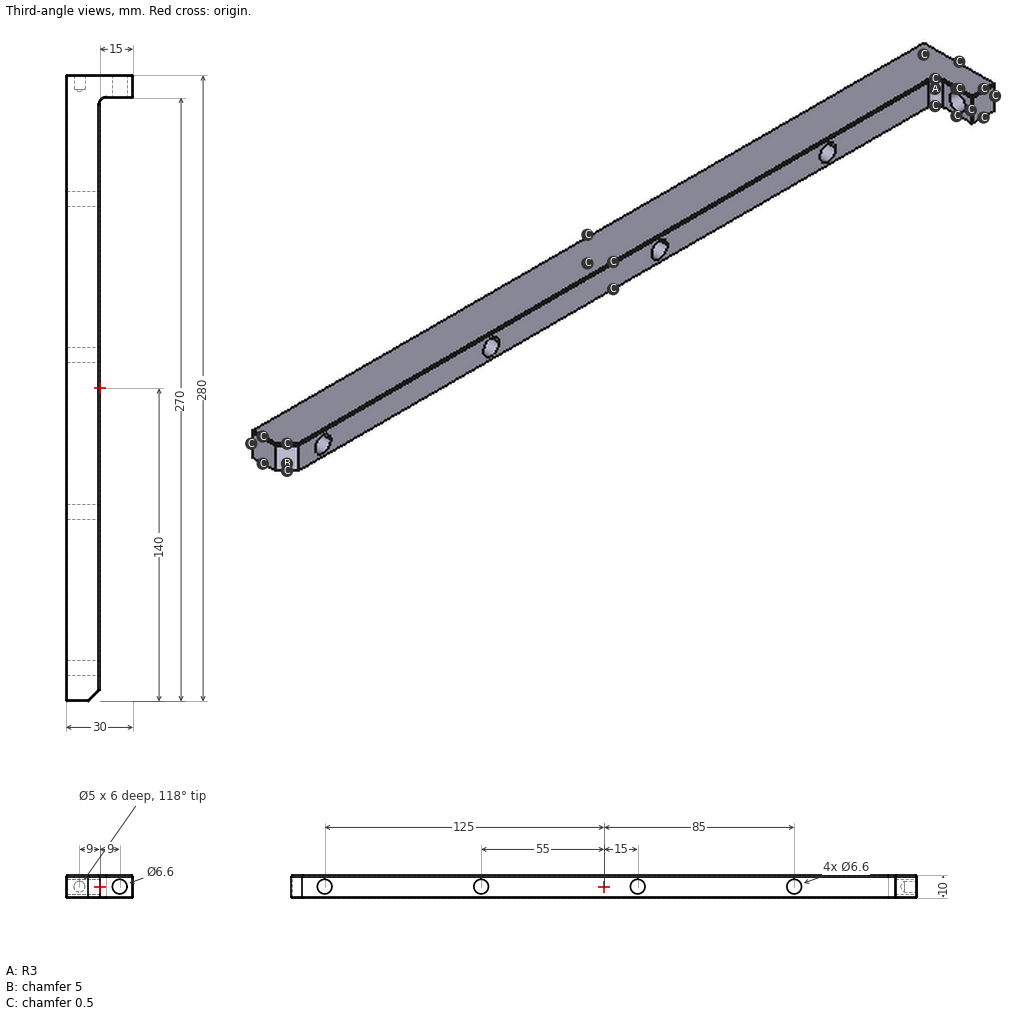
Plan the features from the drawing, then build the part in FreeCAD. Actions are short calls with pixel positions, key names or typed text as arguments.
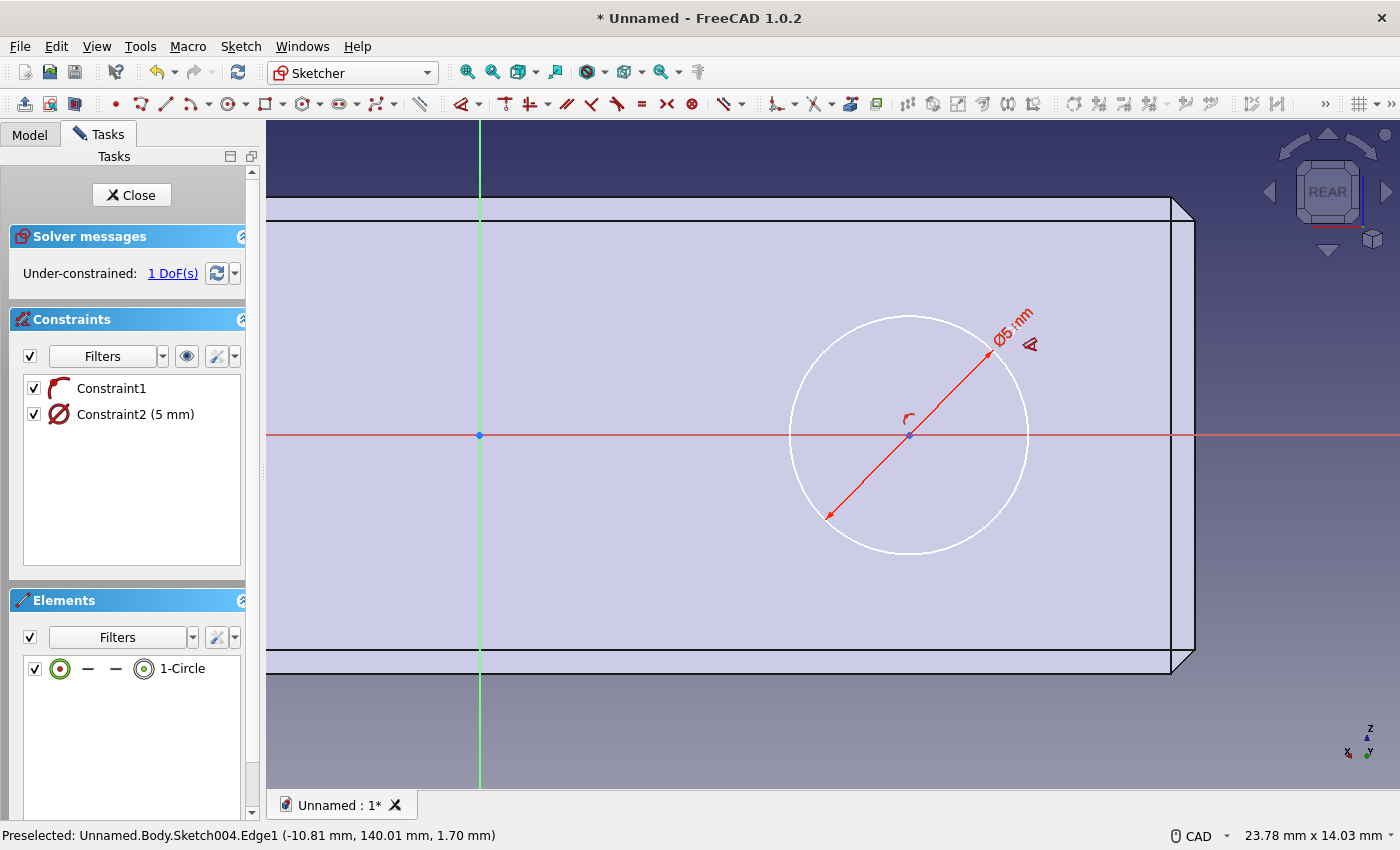
scroll(909, 435, up, 4)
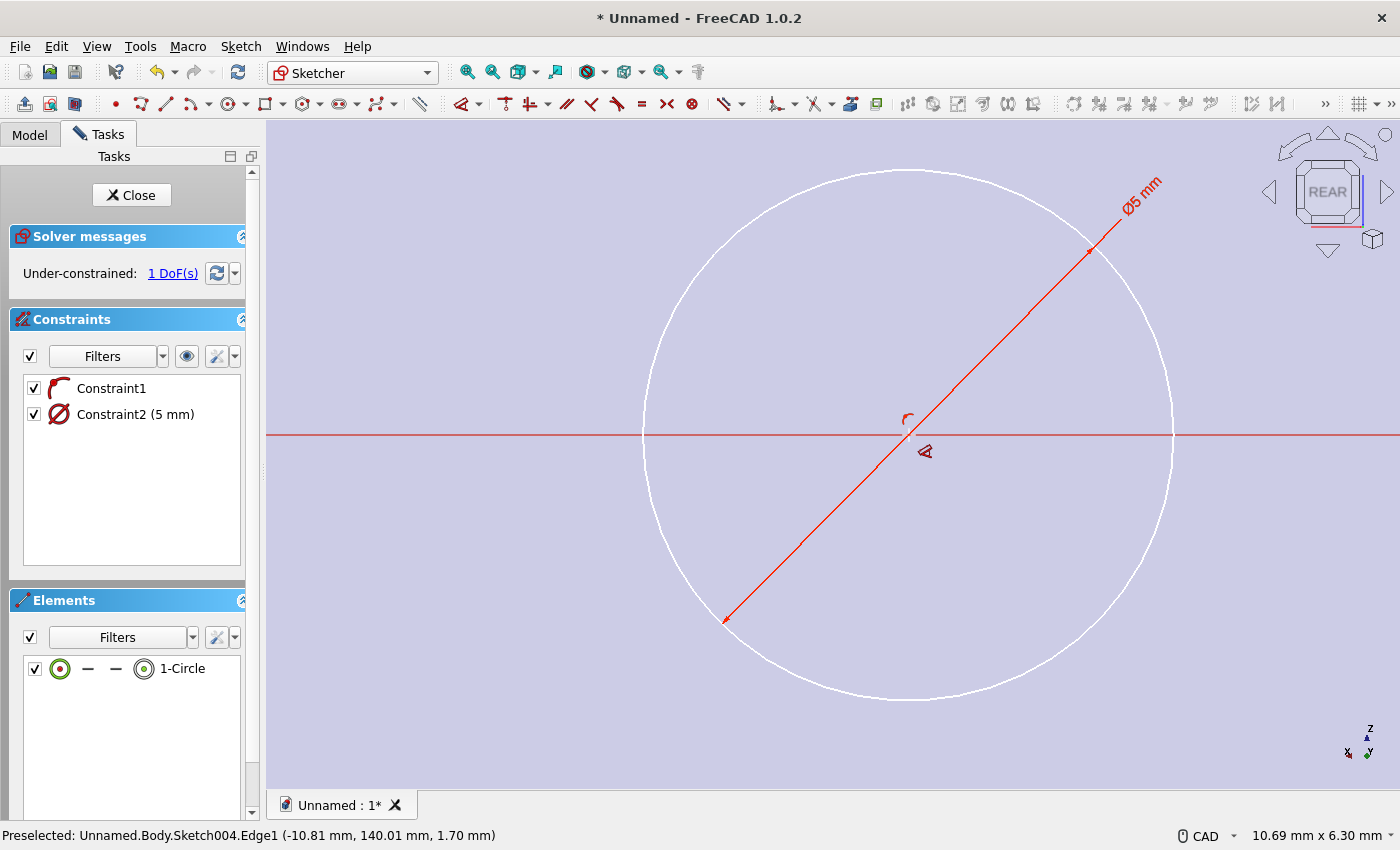
click(908, 435)
click(601, 469)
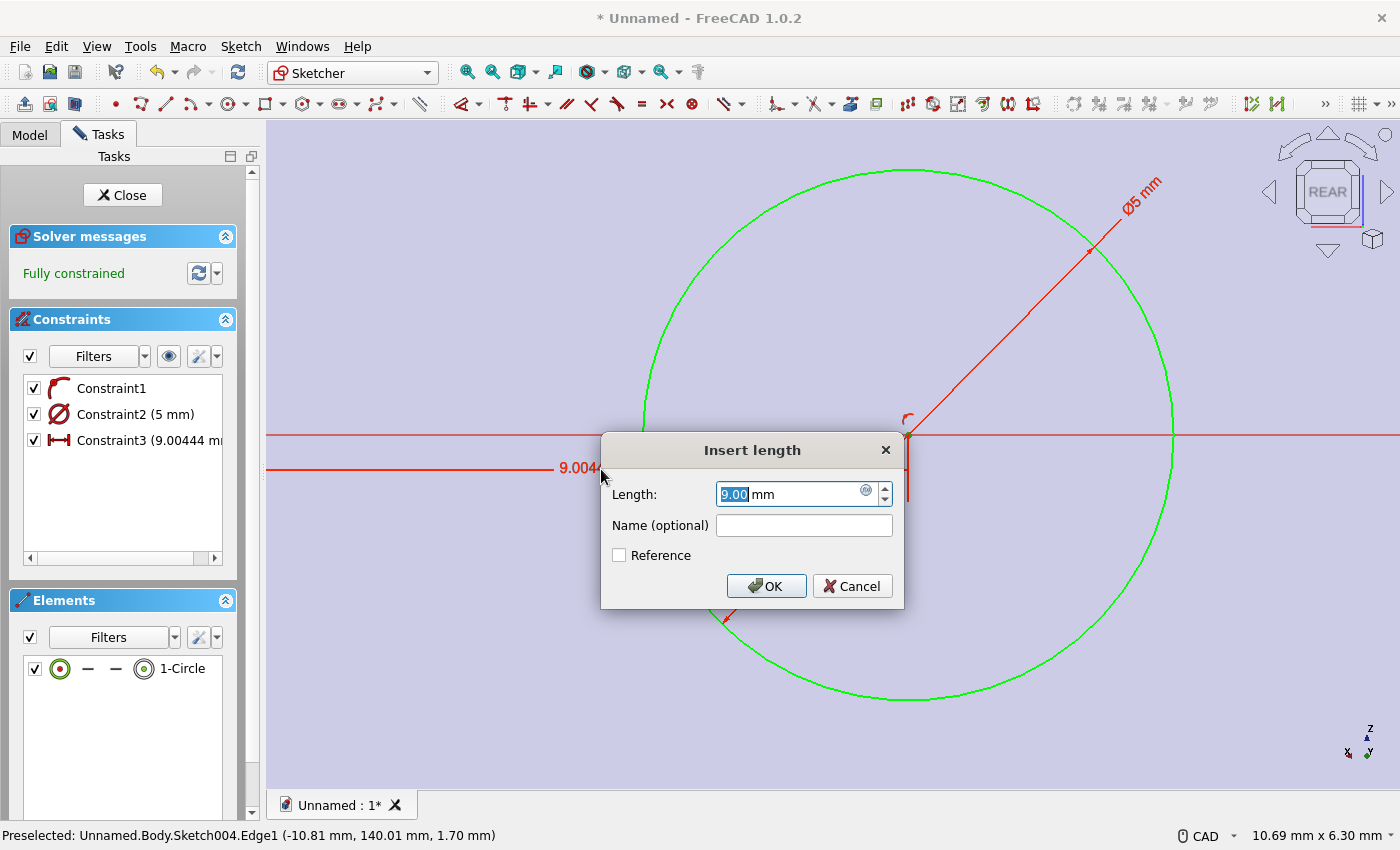
text(9)
key(Return)
key(Escape)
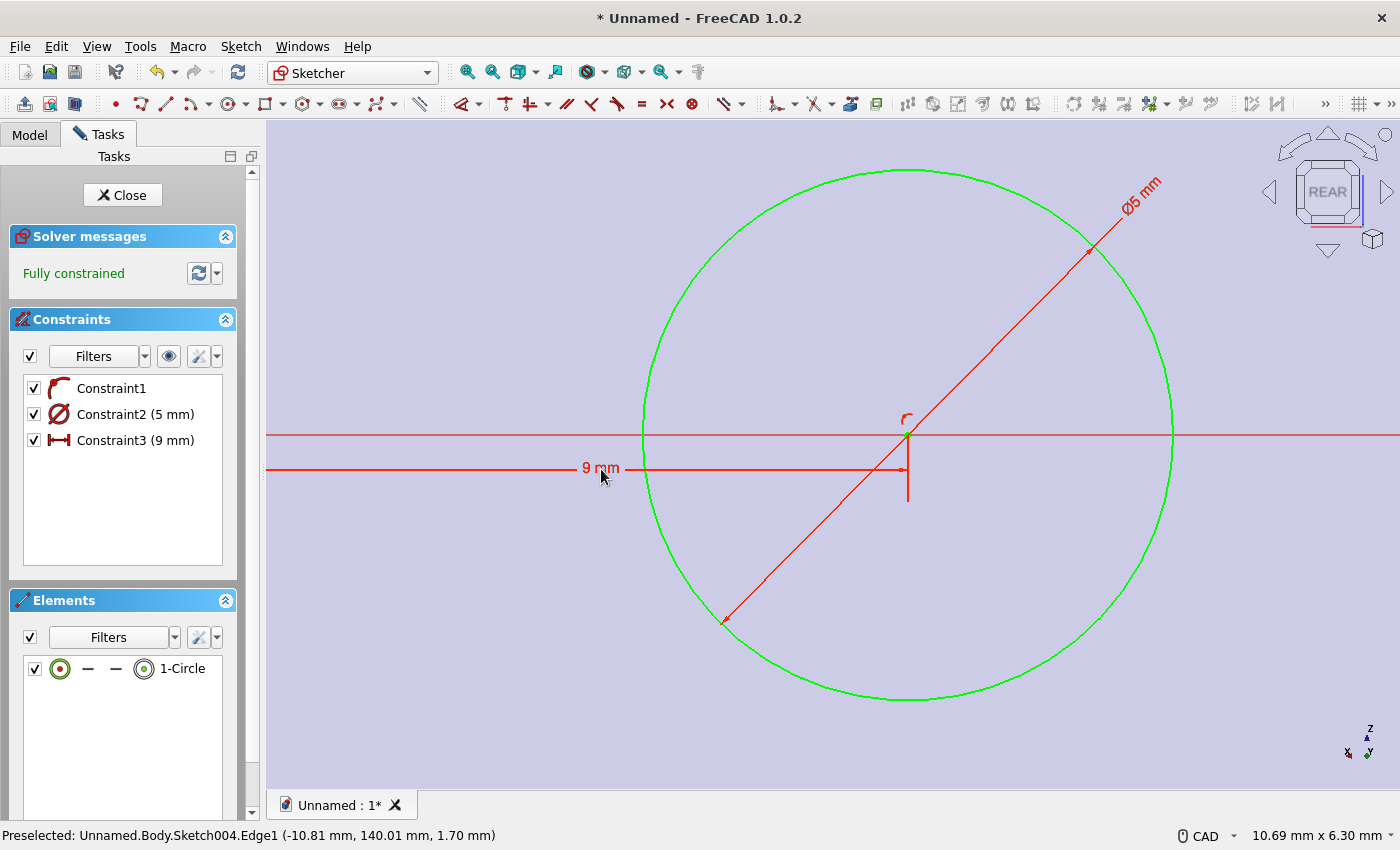
click(123, 195)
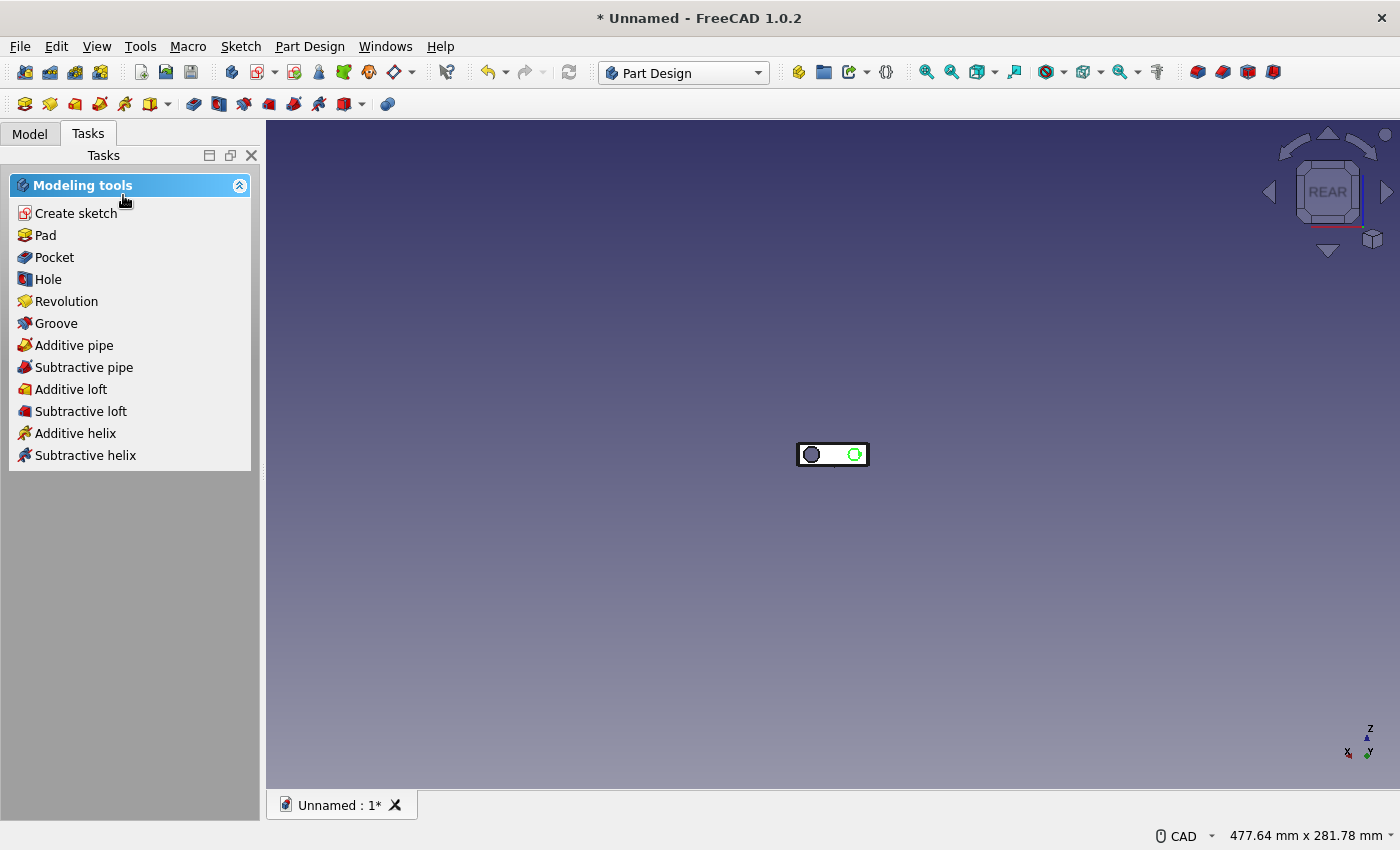
click(219, 104)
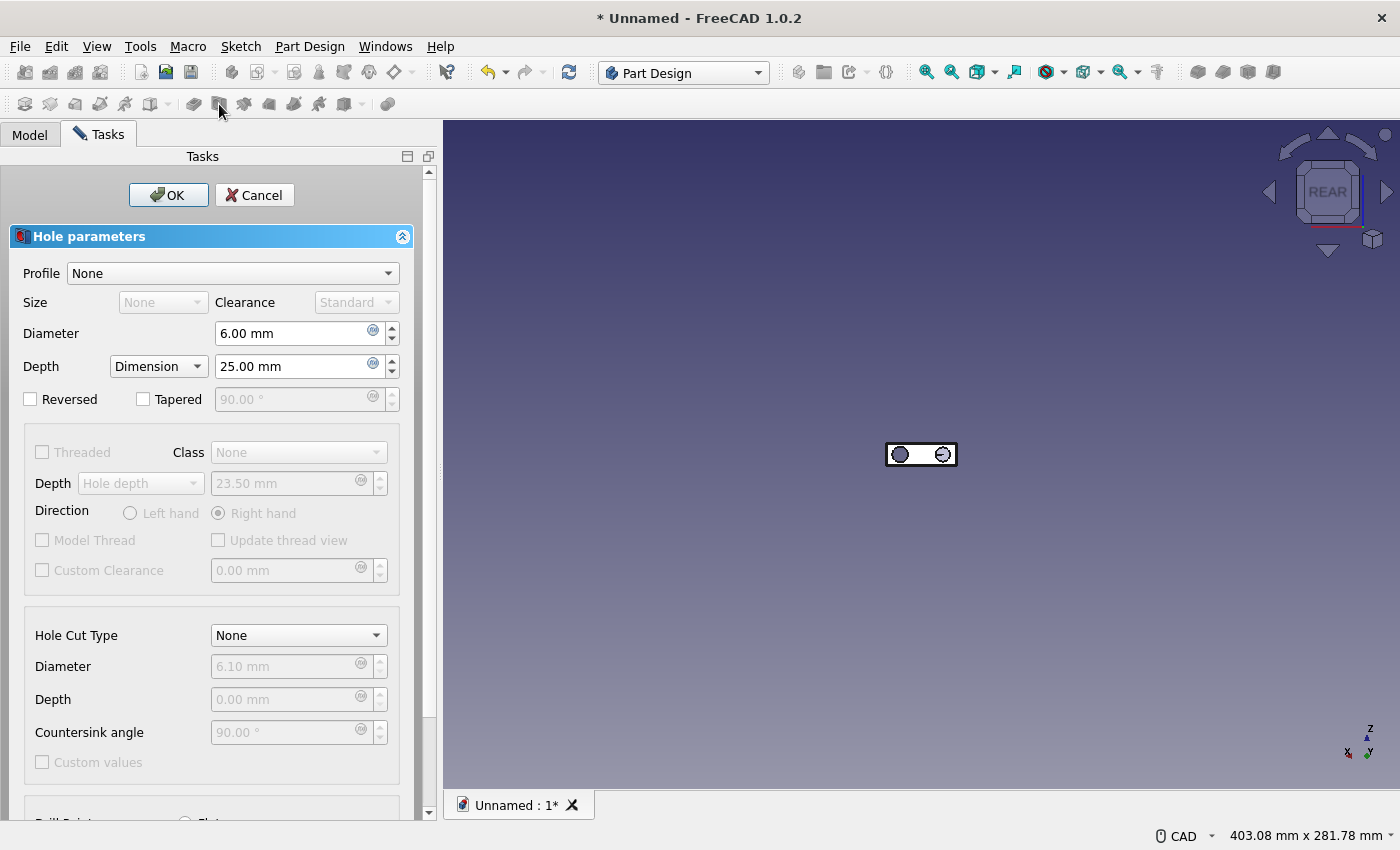
triple_click(300, 334)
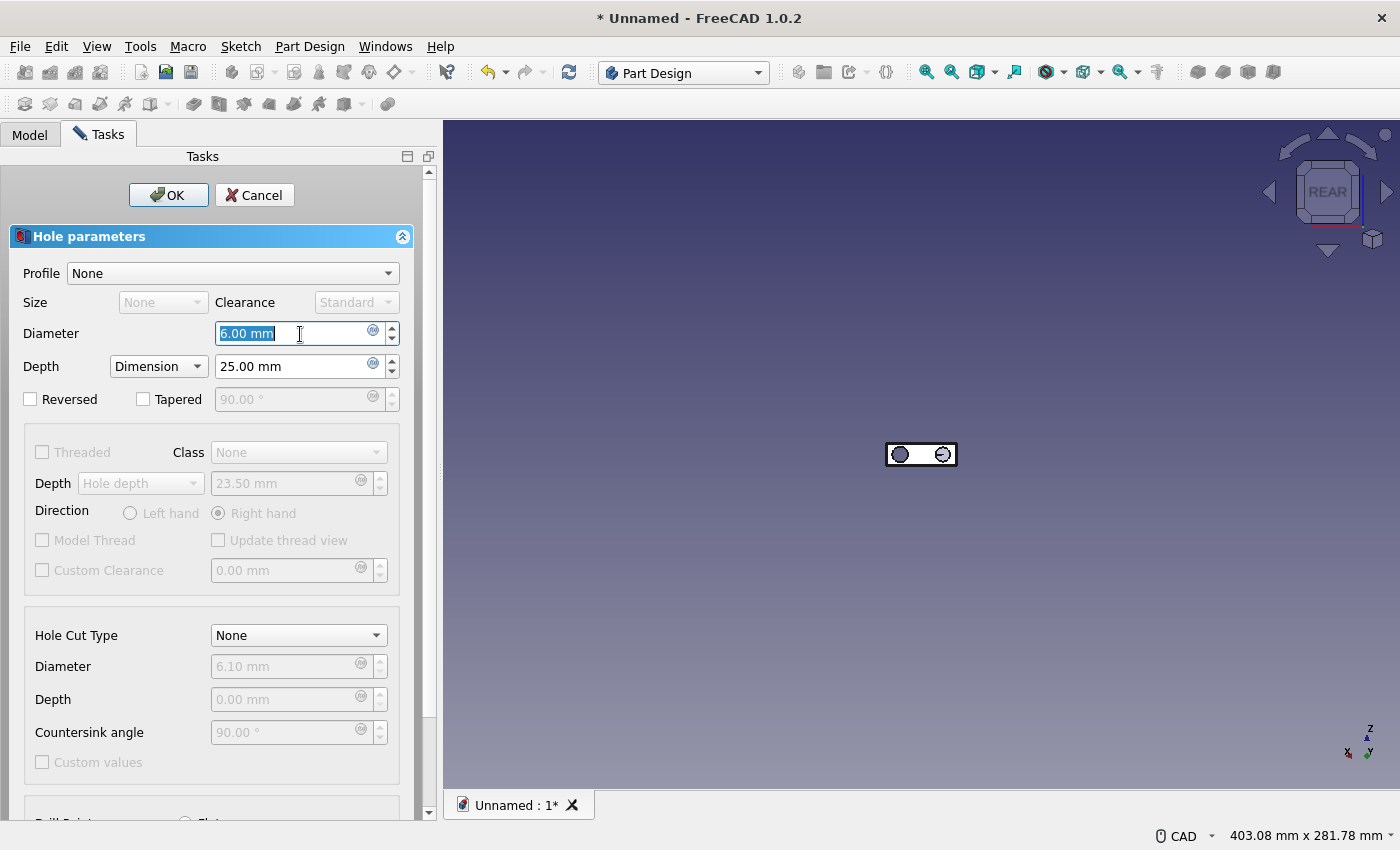
text(5)
key(Tab)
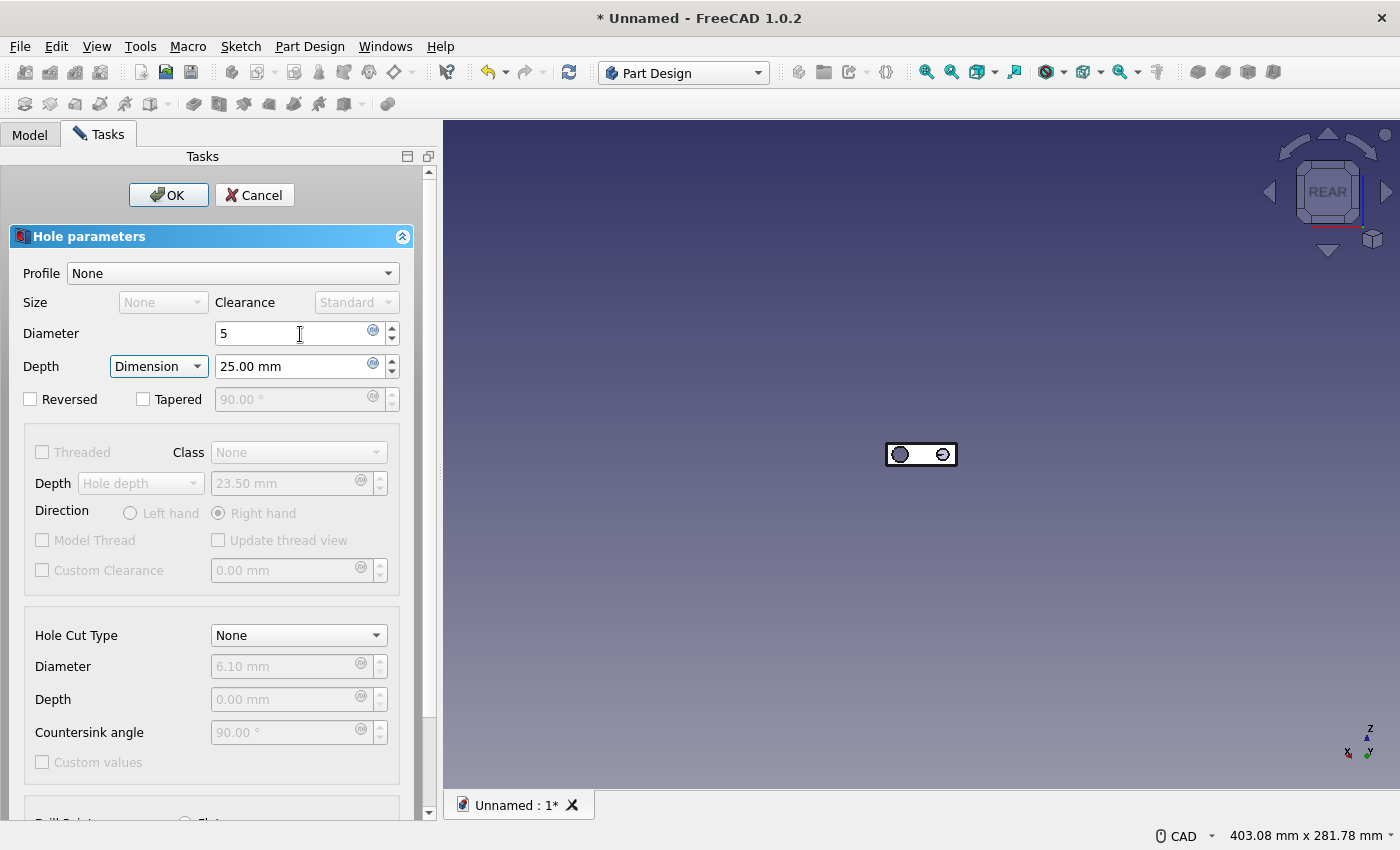
triple_click(300, 366)